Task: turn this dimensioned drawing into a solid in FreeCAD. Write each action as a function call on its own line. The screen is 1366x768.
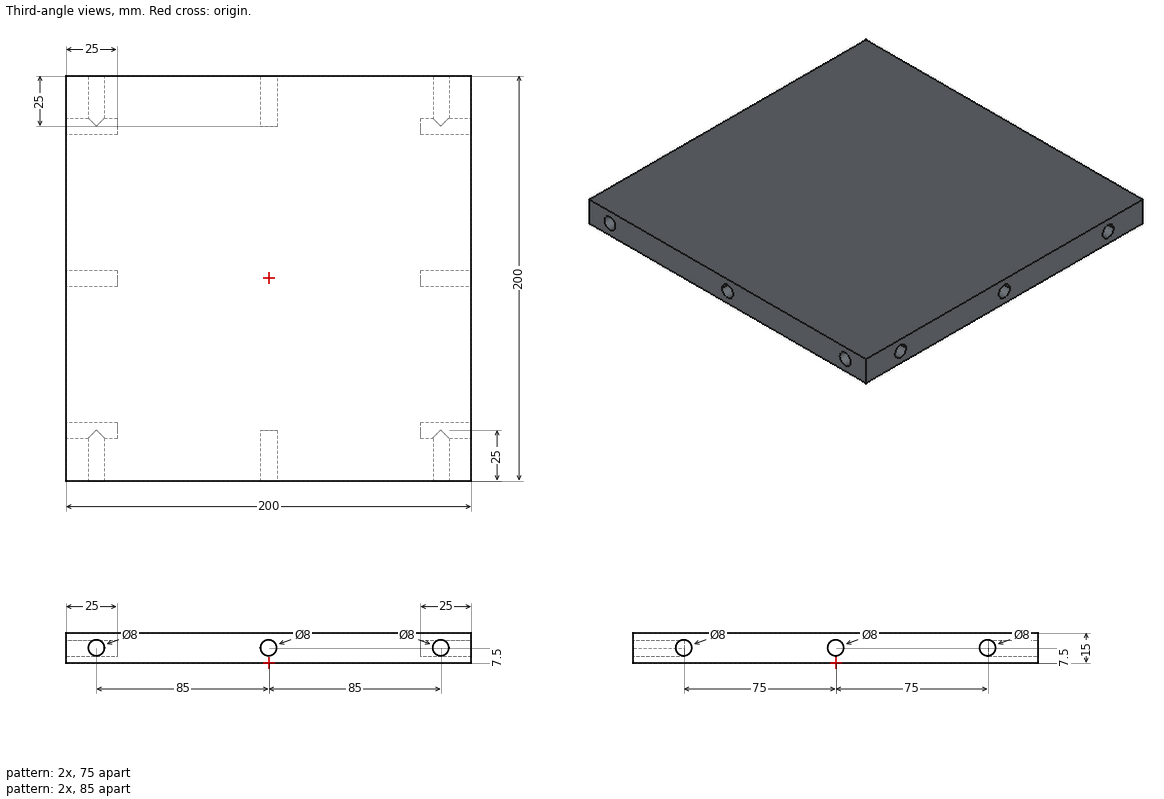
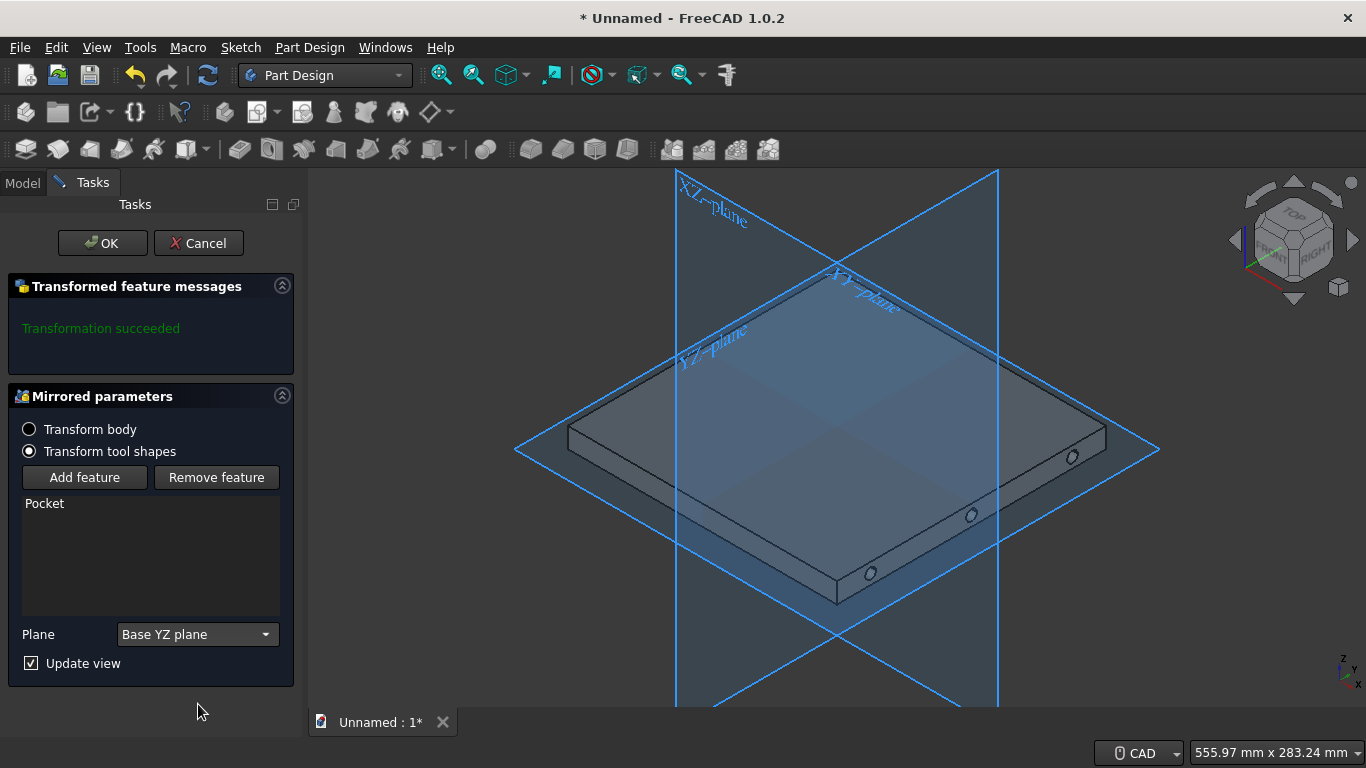
click(103, 243)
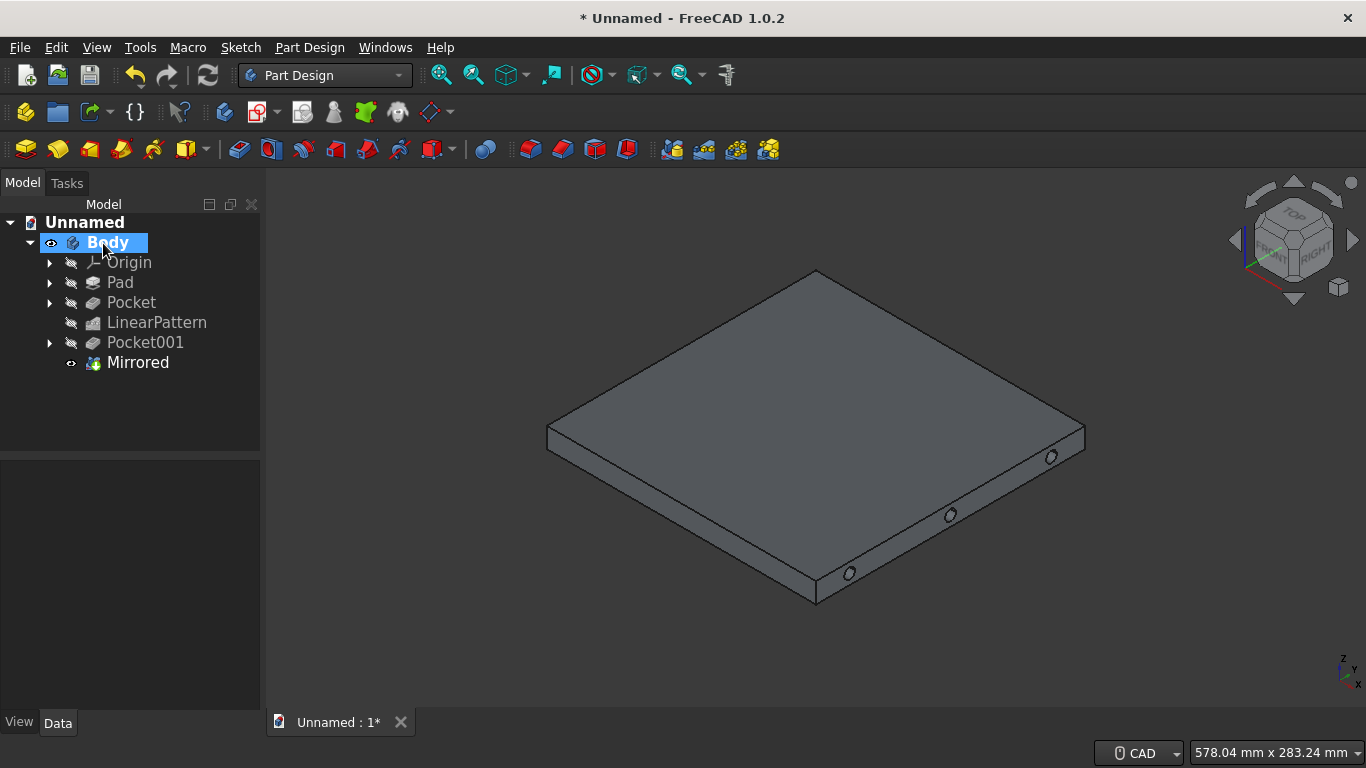
key(6)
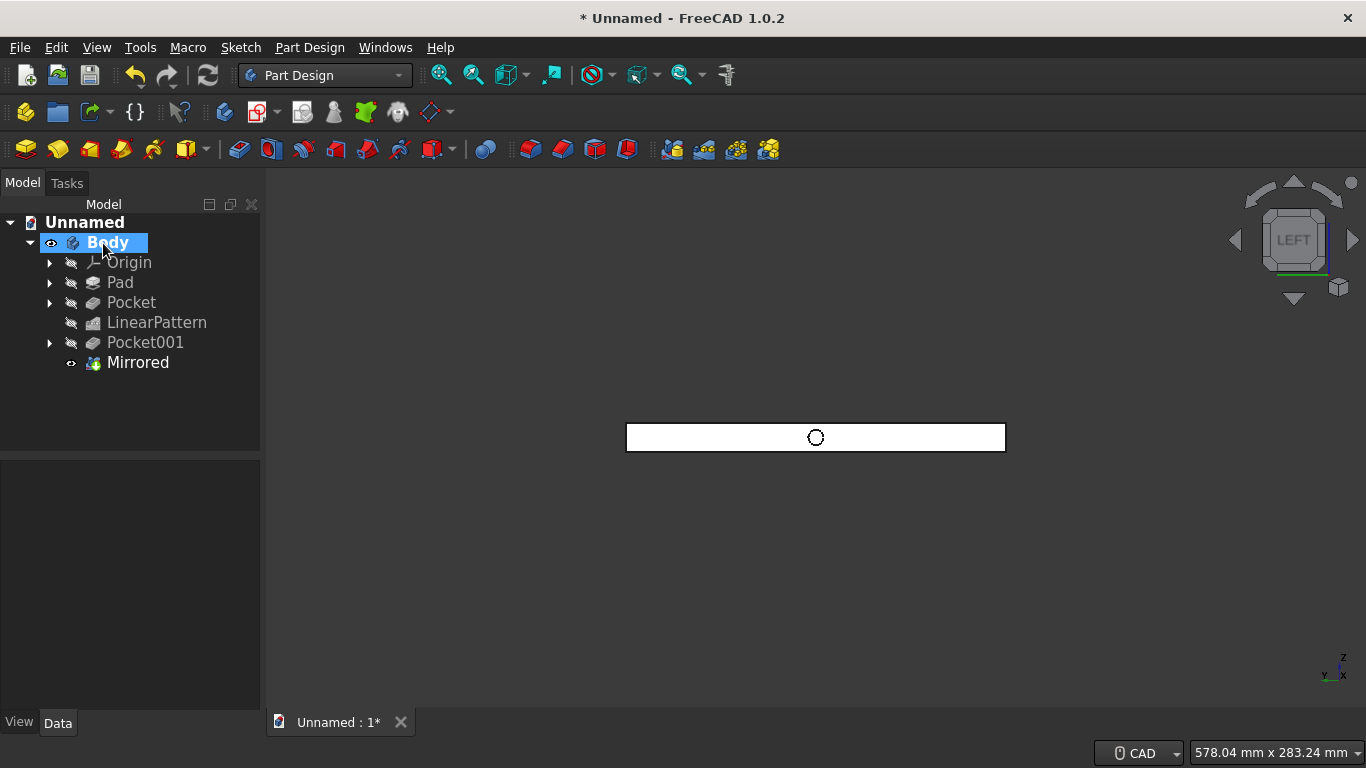
key(v)
key(f)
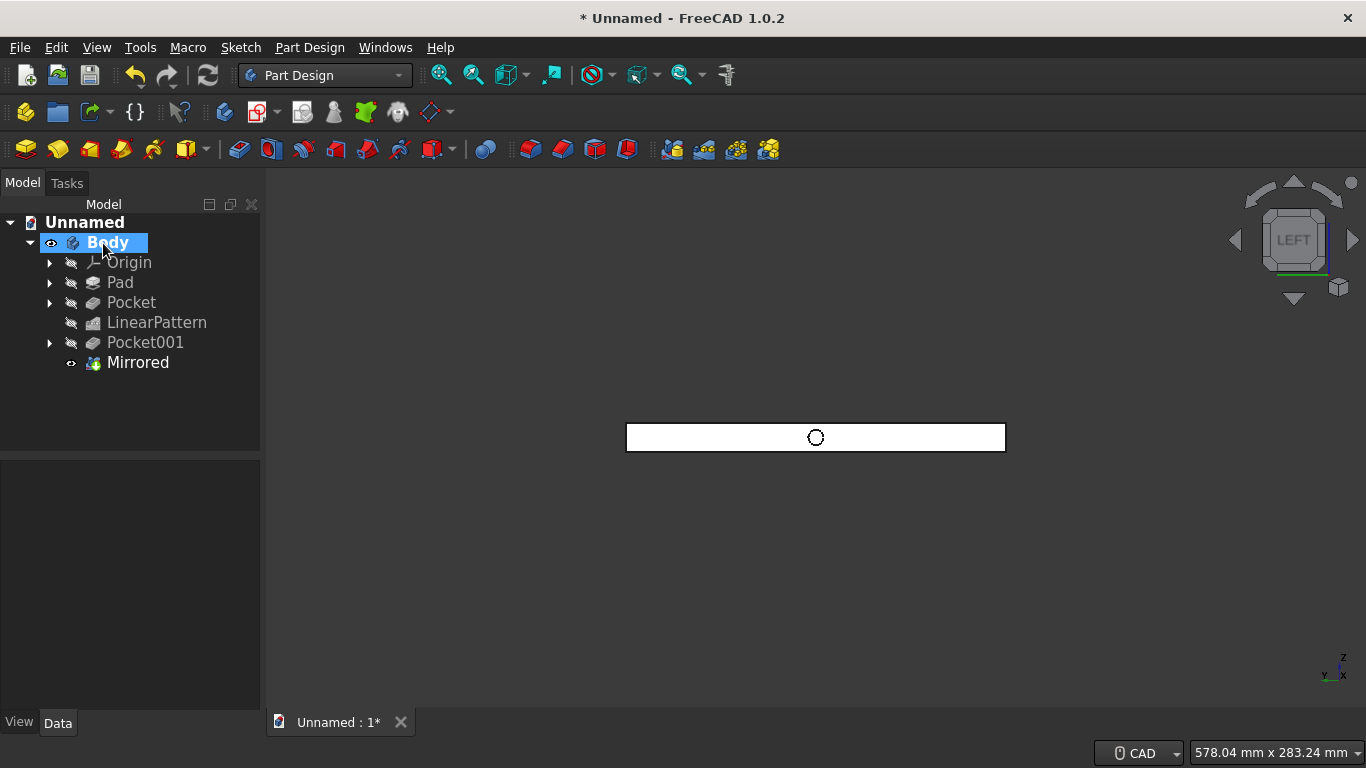
click(653, 436)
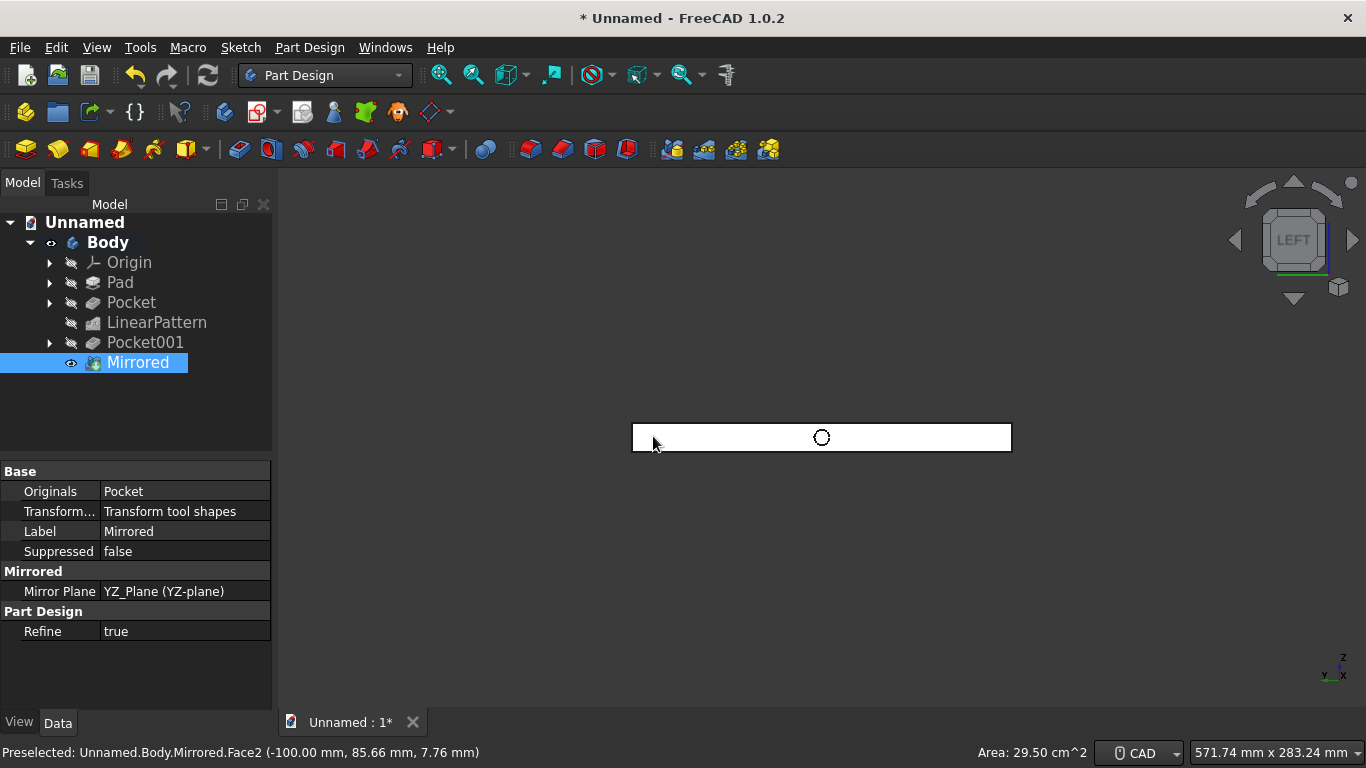
click(258, 112)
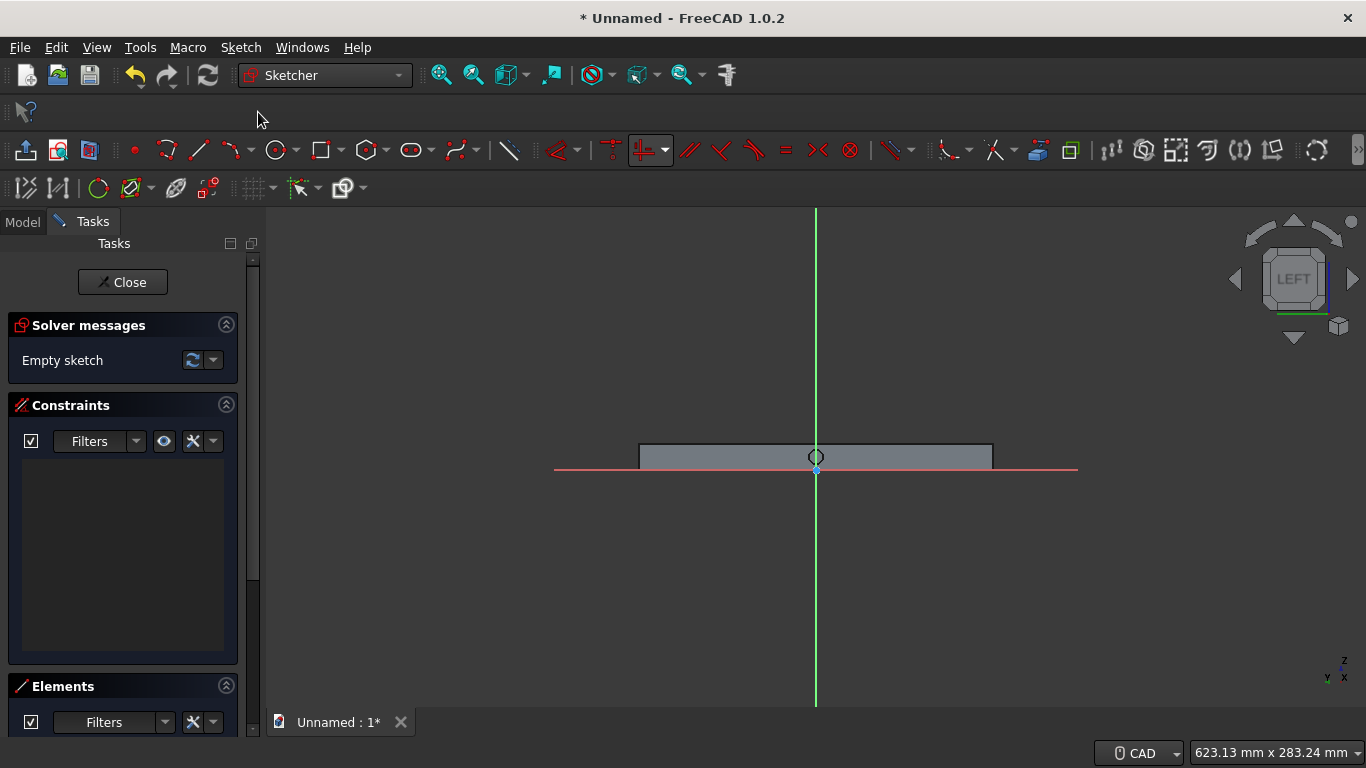
scroll(959, 457, up, 15)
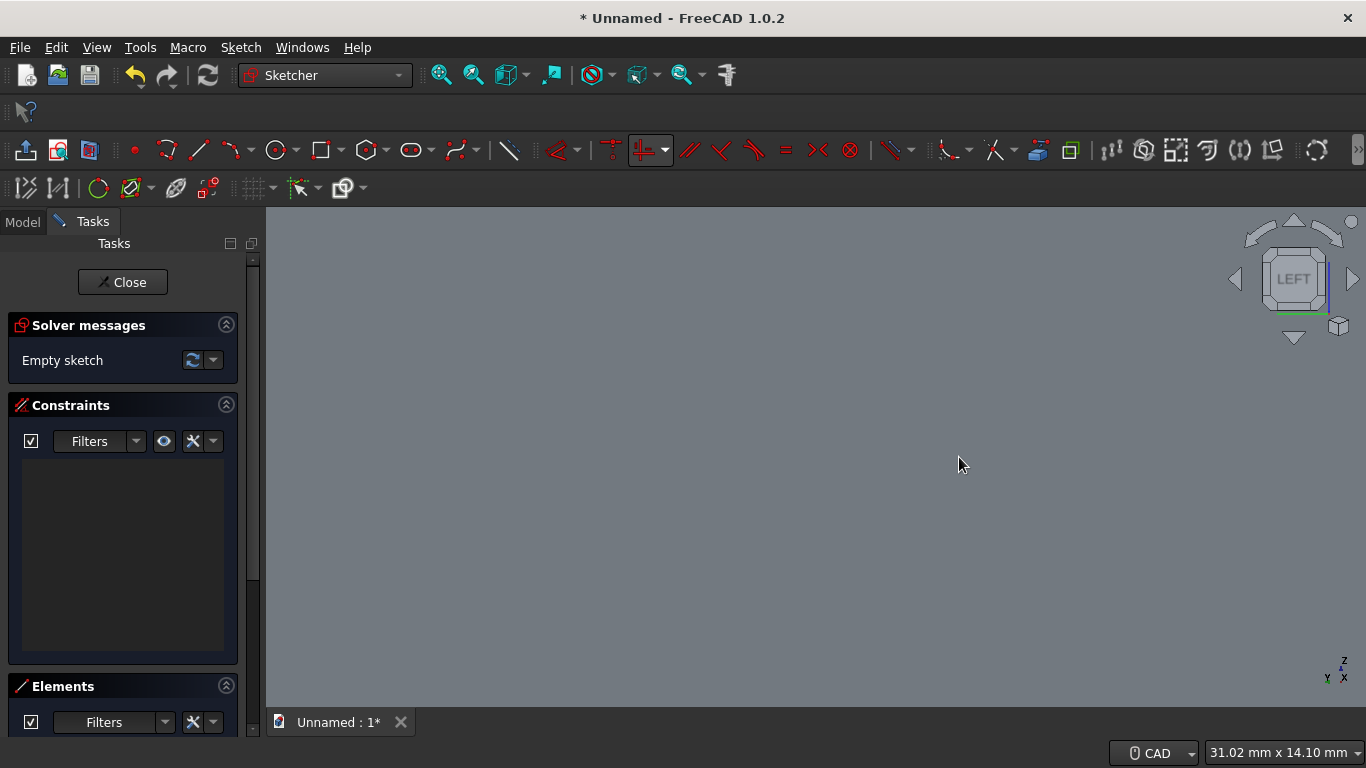
click(276, 150)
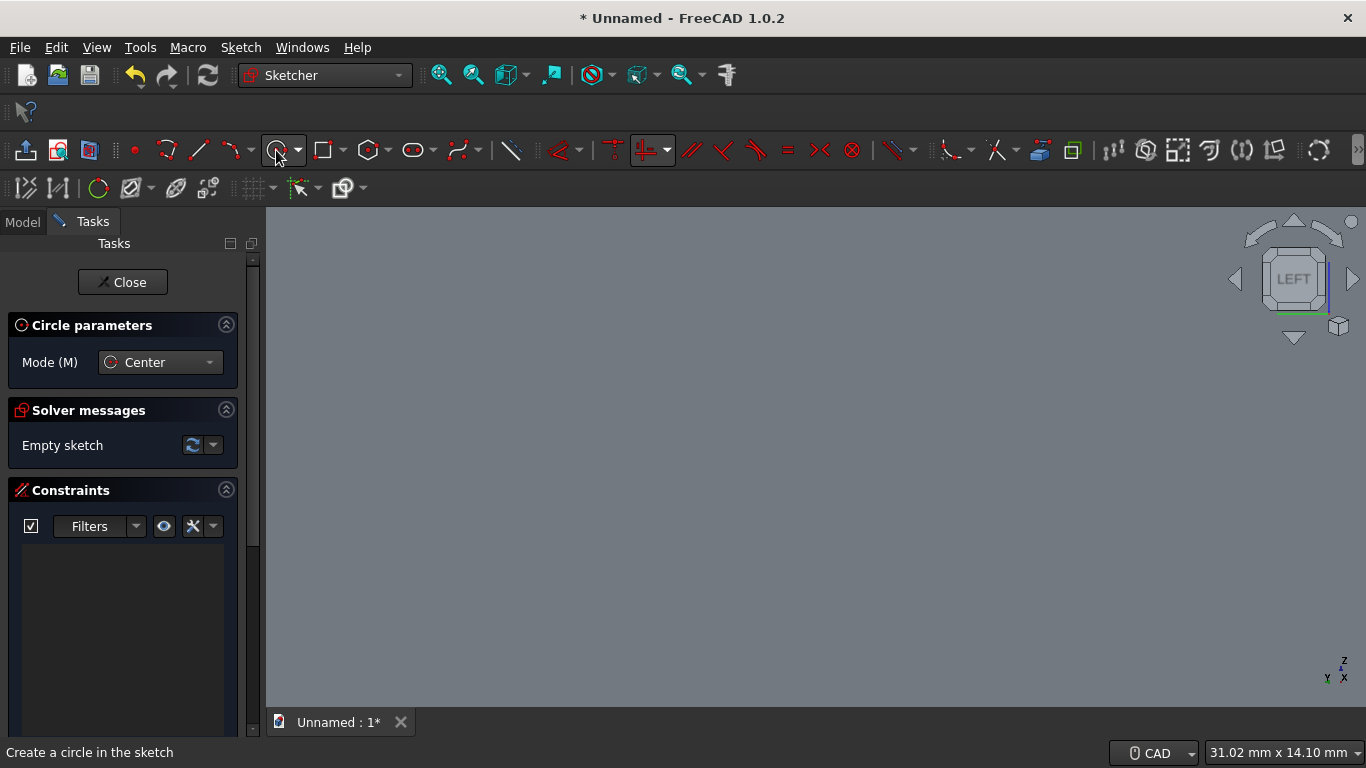
click(734, 447)
move(834, 347)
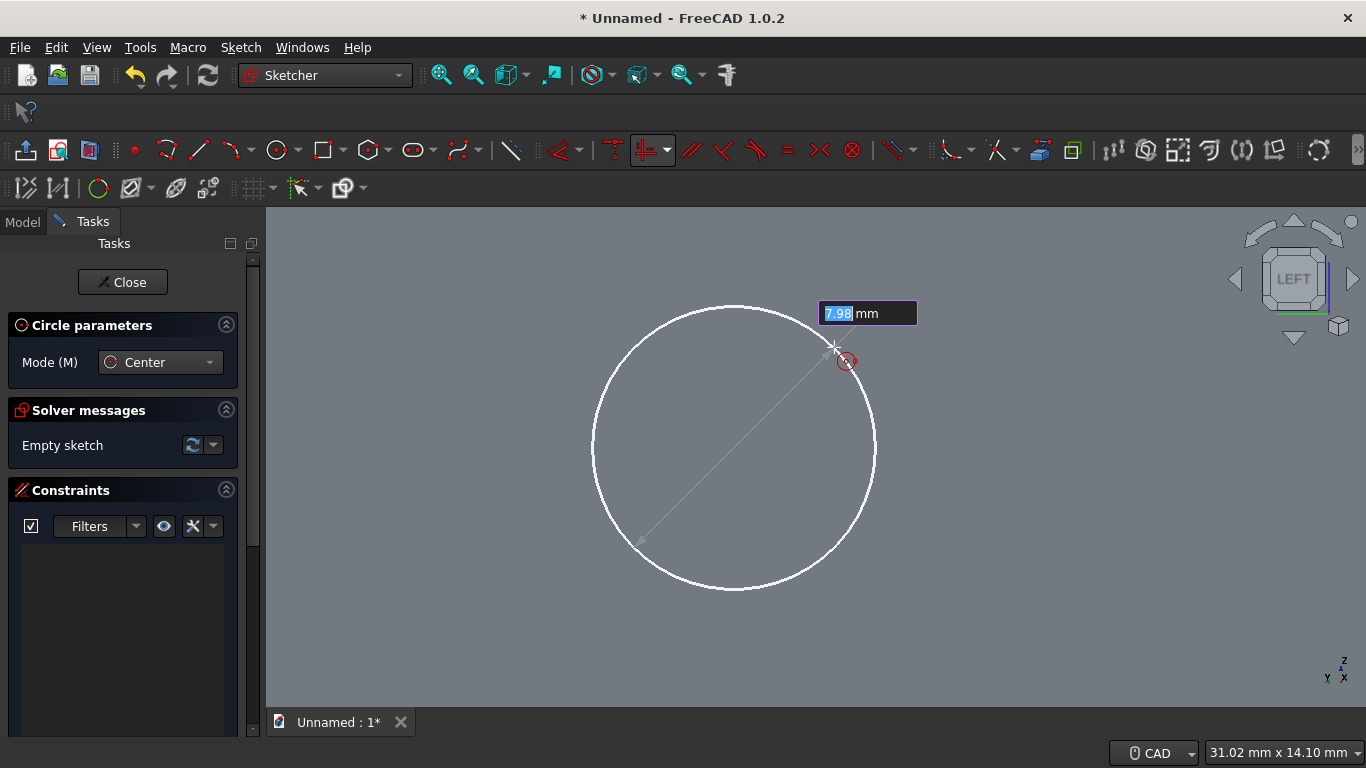
text(8)
key(Return)
key(Escape)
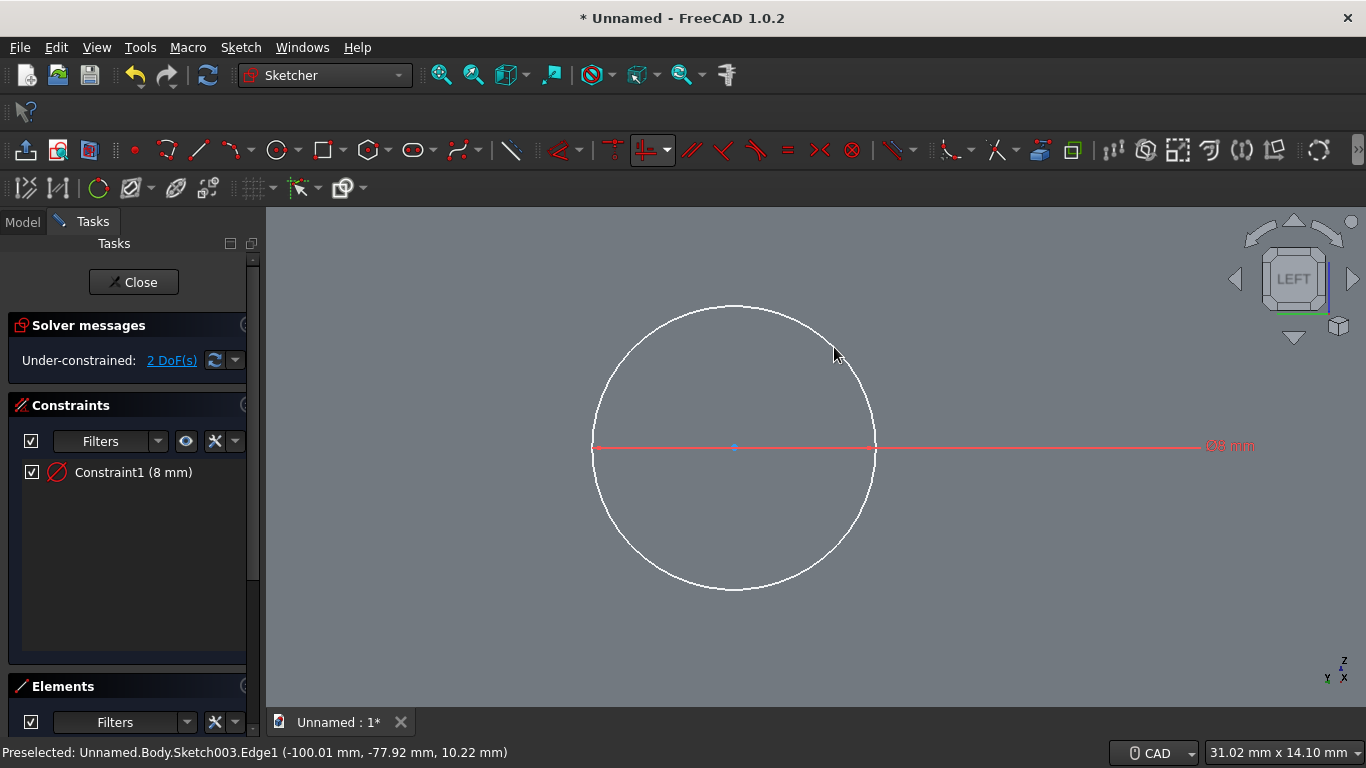
key(d)